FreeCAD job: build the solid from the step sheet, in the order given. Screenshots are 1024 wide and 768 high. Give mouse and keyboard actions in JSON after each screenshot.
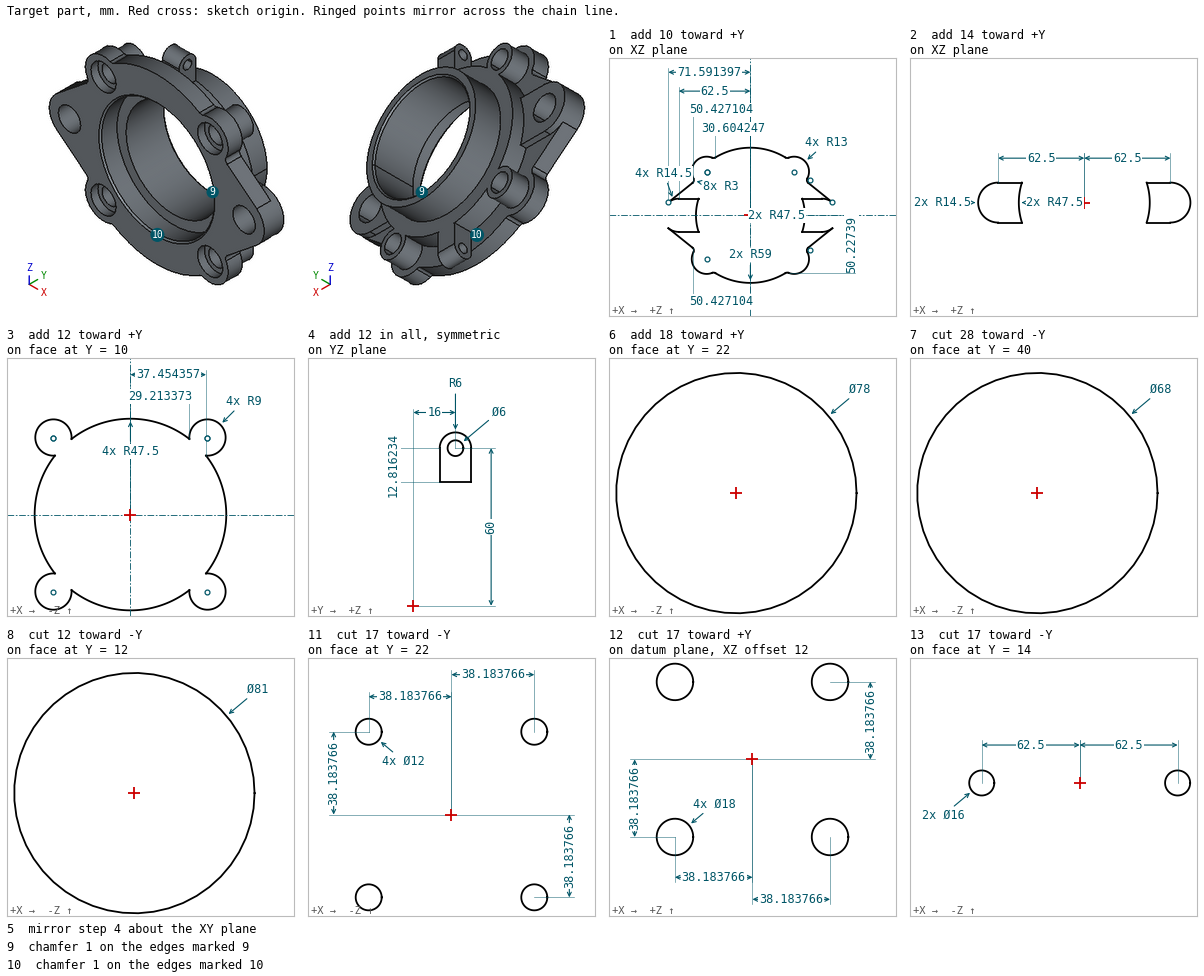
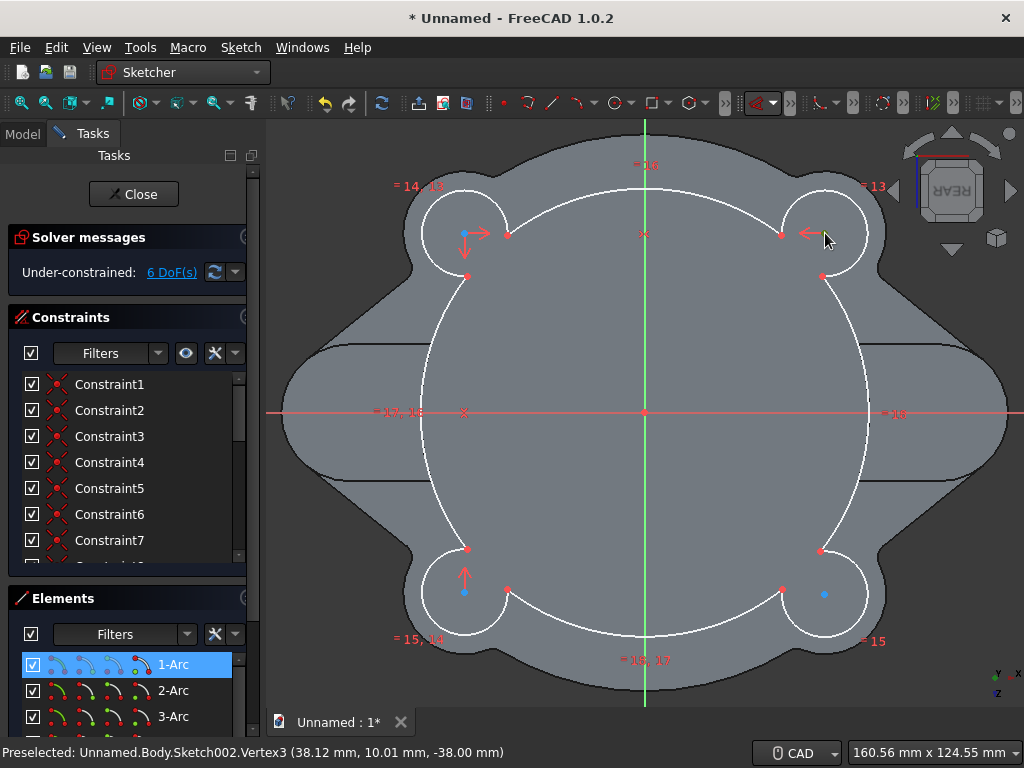
{"action": "left_click", "coordinate": [825, 594]}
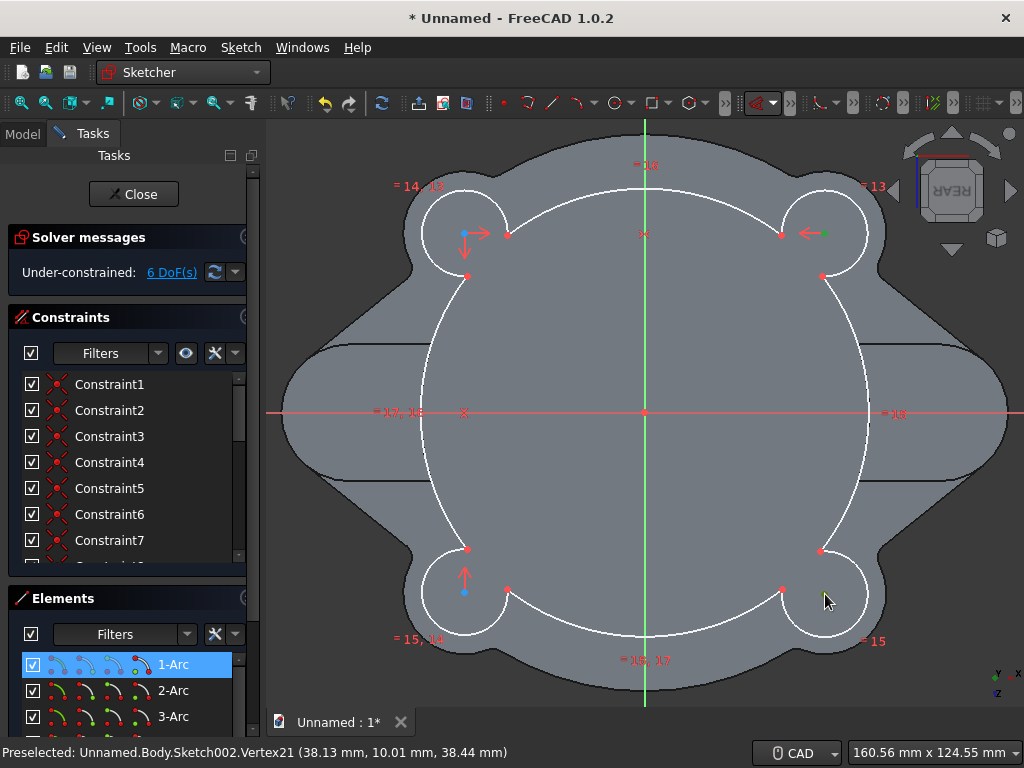
{"action": "left_click", "coordinate": [334, 413]}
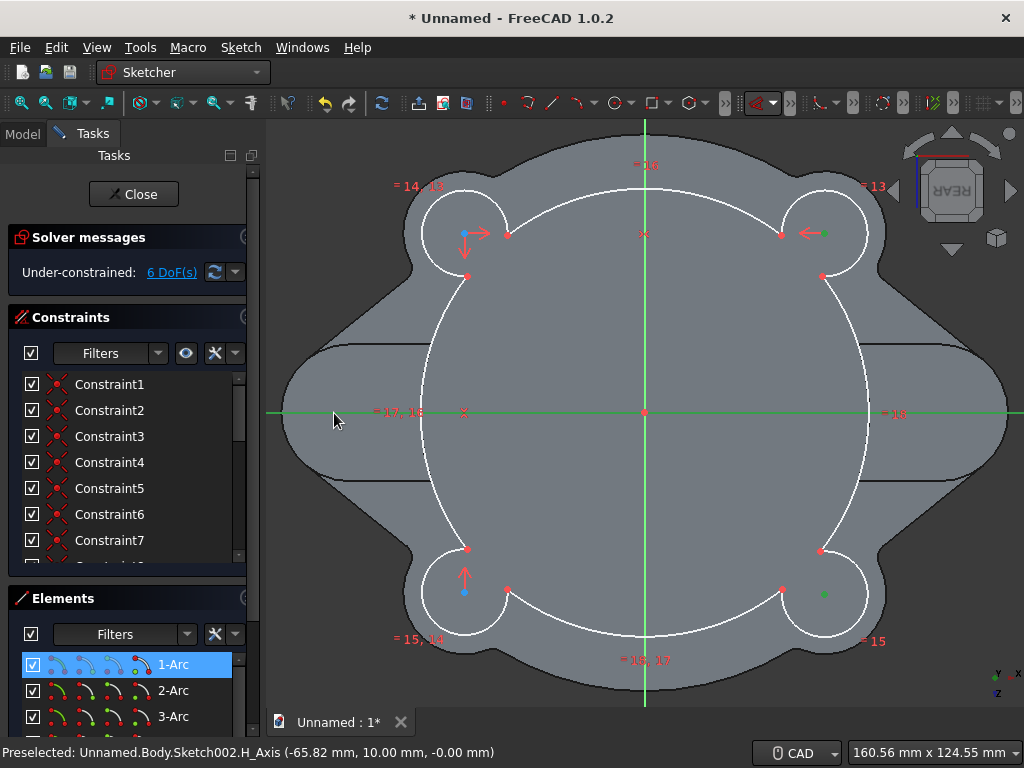
{"action": "key", "text": "s"}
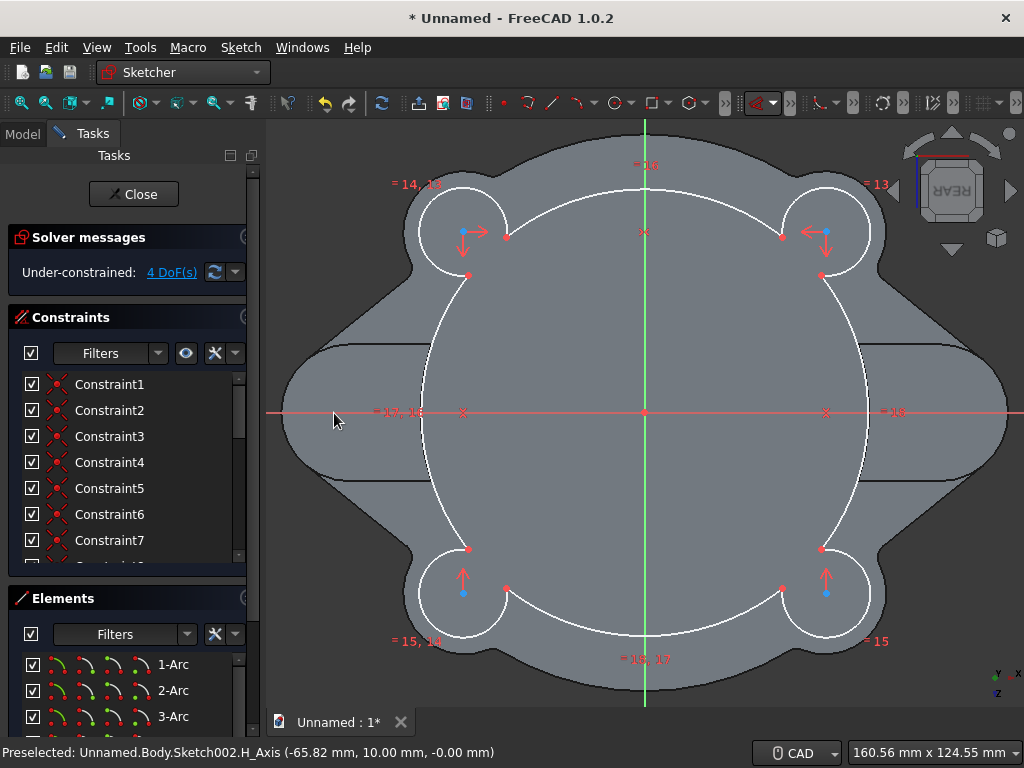
{"action": "key", "text": "d"}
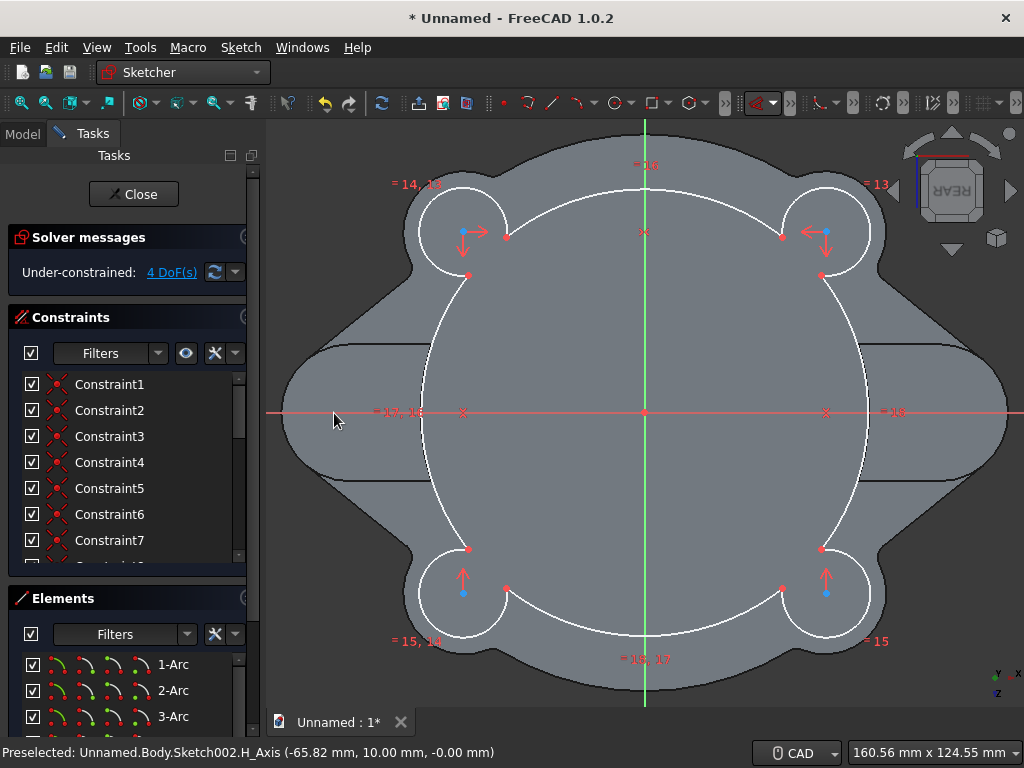
{"action": "left_click", "coordinate": [817, 189]}
{"action": "left_click", "coordinate": [810, 158]}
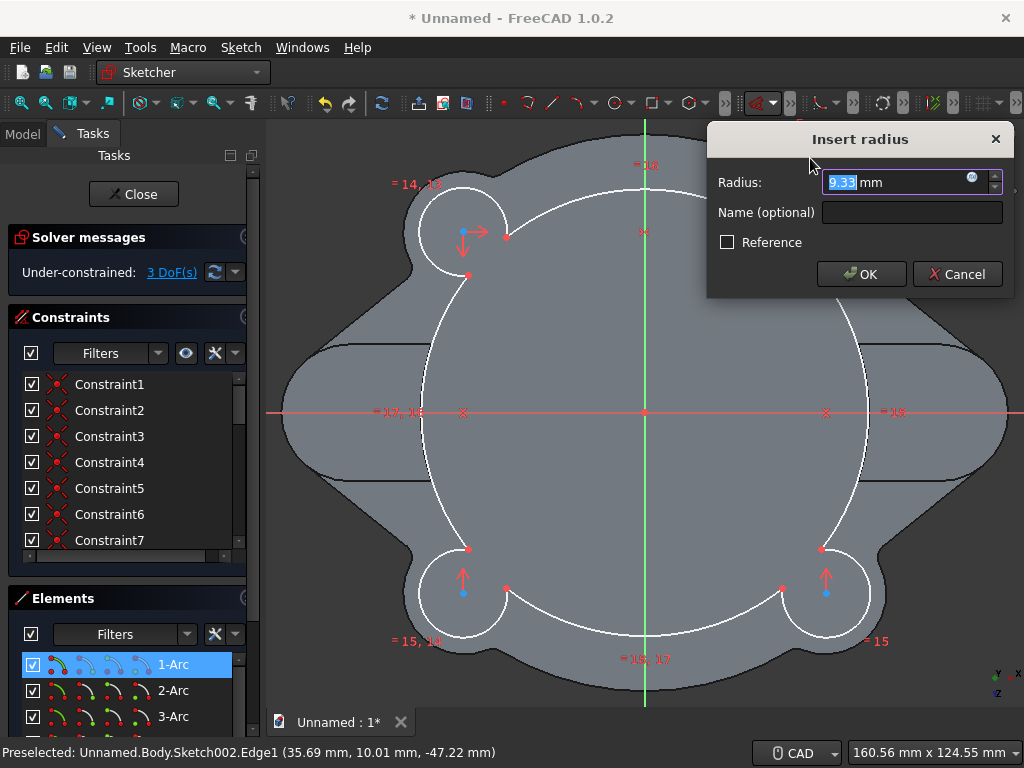
{"action": "type", "text": "9"}
{"action": "key", "text": "Return"}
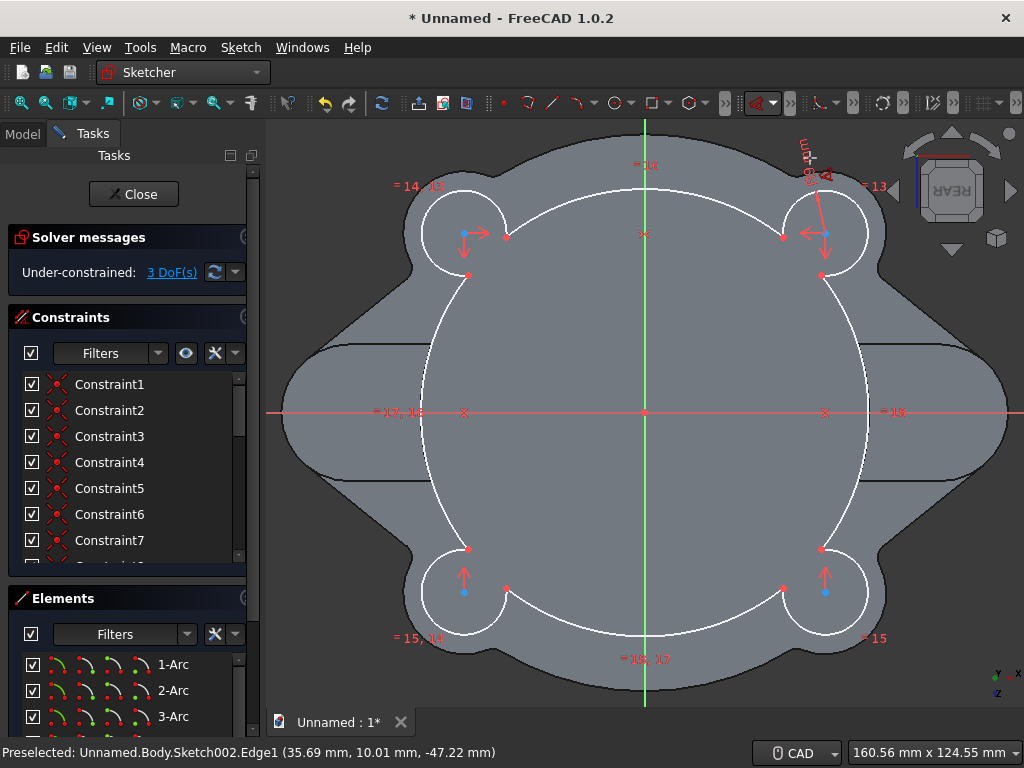
{"action": "left_click", "coordinate": [704, 197]}
{"action": "left_click", "coordinate": [712, 166]}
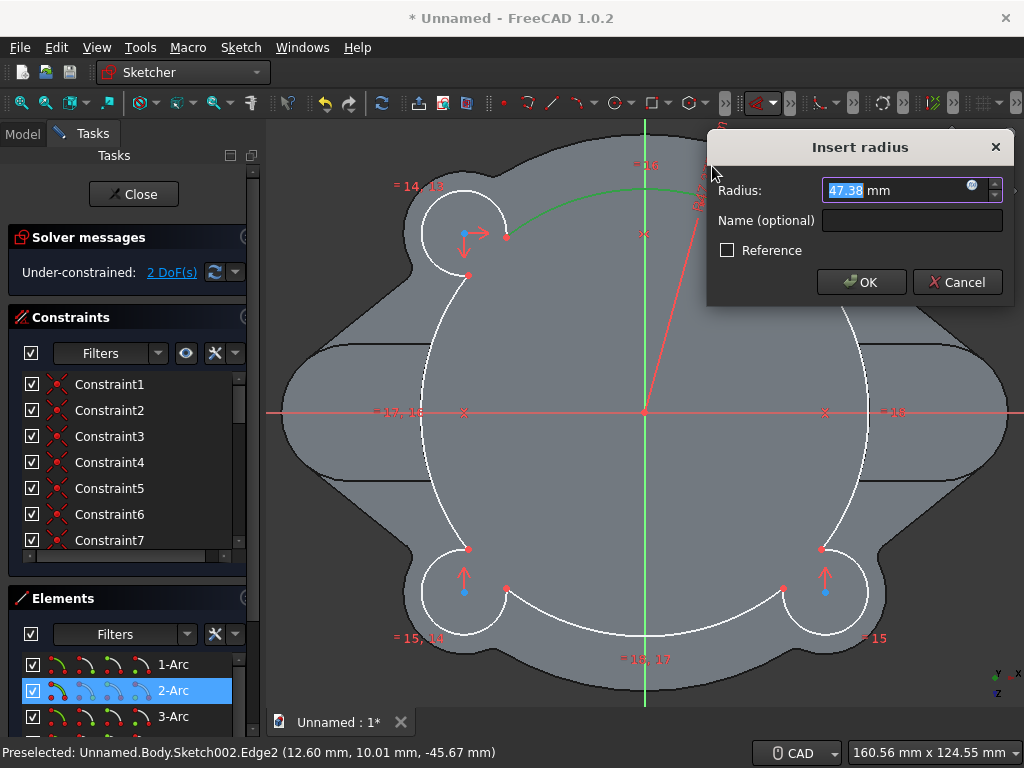
{"action": "type", "text": "47.5"}
{"action": "key", "text": "Return"}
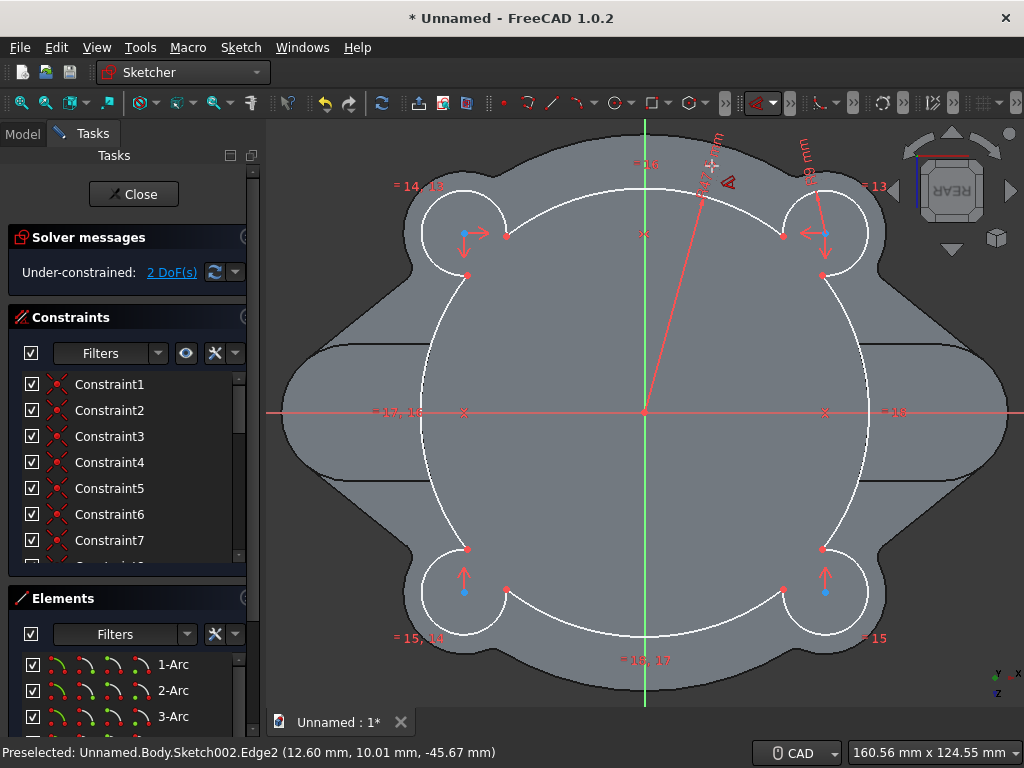
{"action": "left_click", "coordinate": [822, 276]}
{"action": "left_click", "coordinate": [733, 242]}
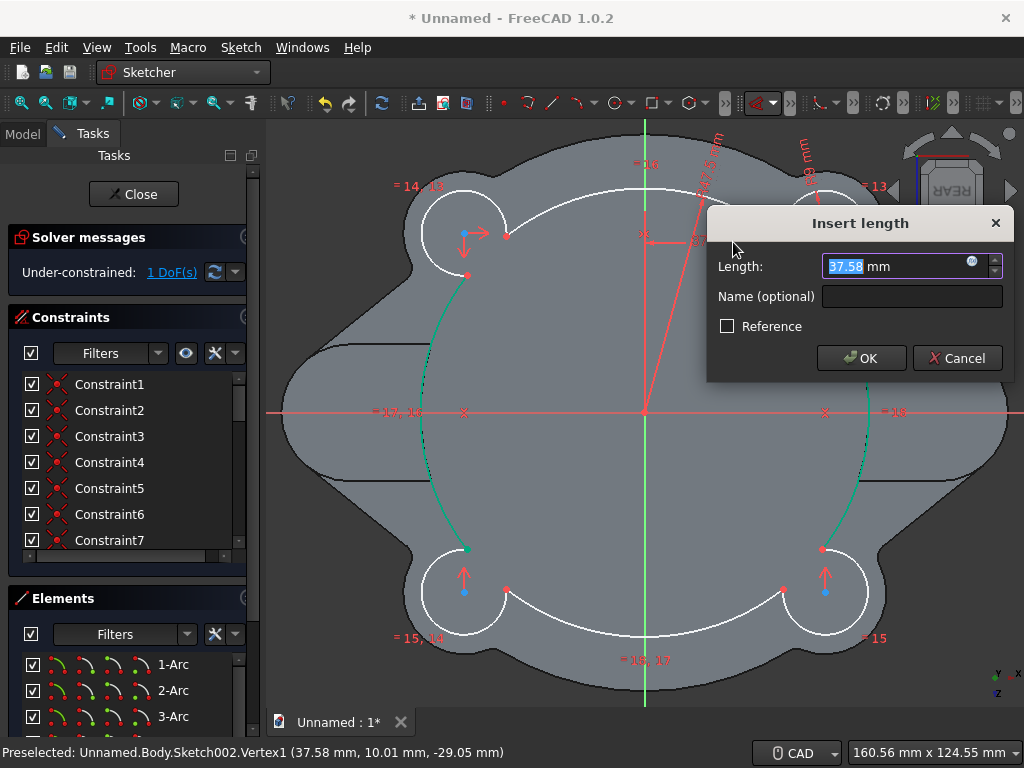
{"action": "type", "text": "37.454357"}
{"action": "key", "text": "Return"}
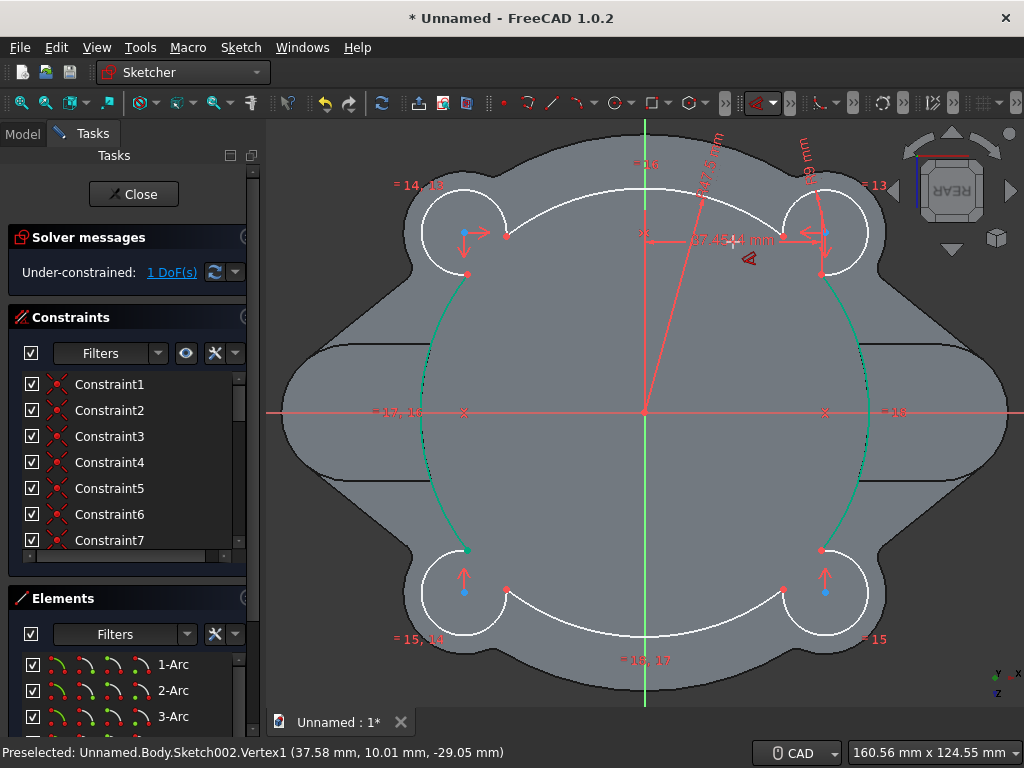
{"action": "left_click", "coordinate": [783, 236]}
{"action": "left_click", "coordinate": [762, 202]}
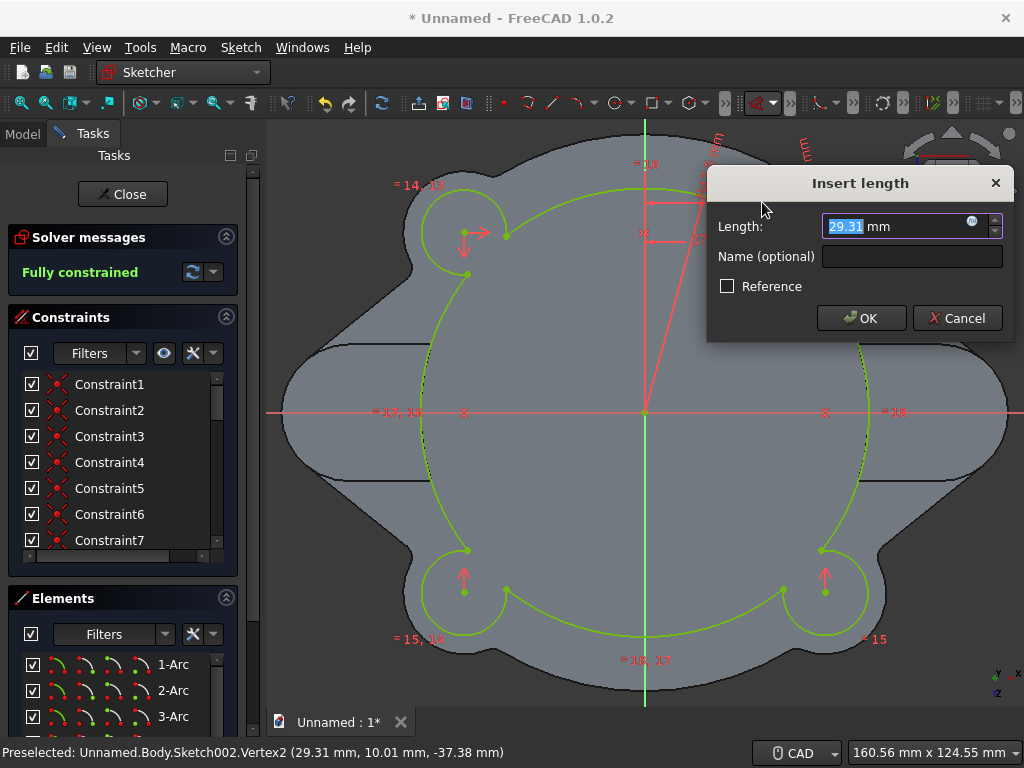
{"action": "type", "text": "29.213373"}
{"action": "key", "text": "Return"}
{"action": "key", "text": "Escape"}